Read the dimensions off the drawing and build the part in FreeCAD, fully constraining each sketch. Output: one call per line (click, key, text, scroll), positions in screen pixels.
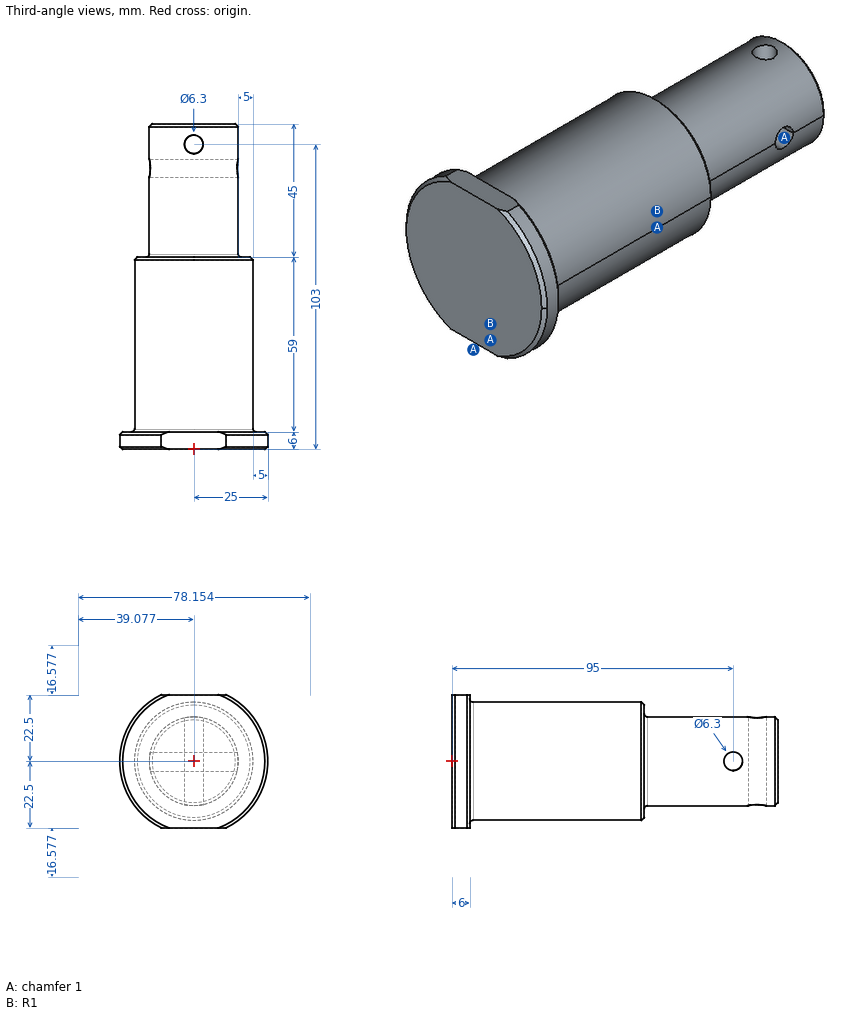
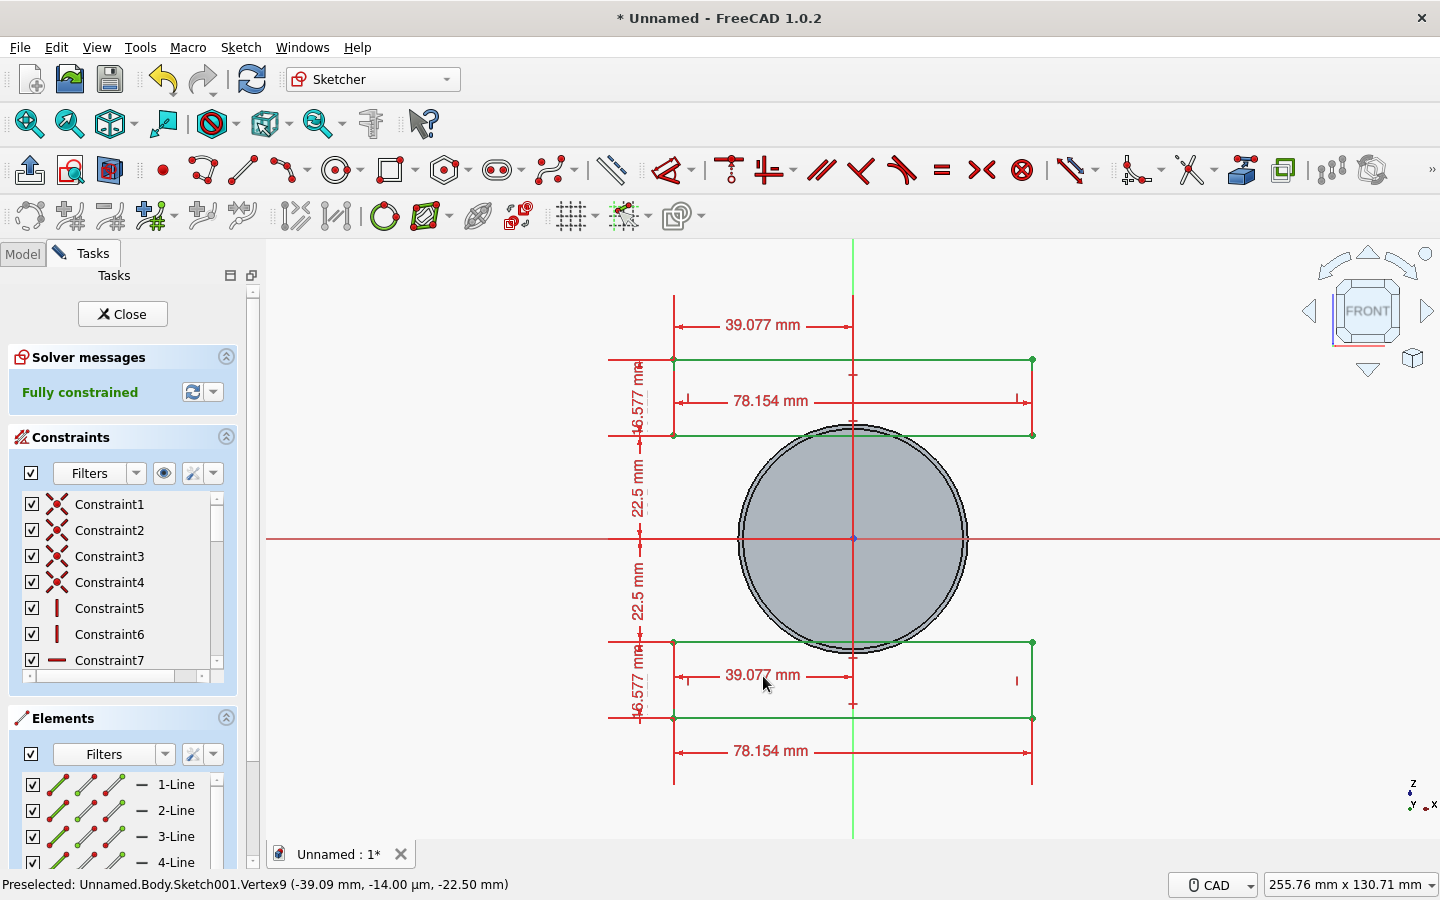
click(123, 314)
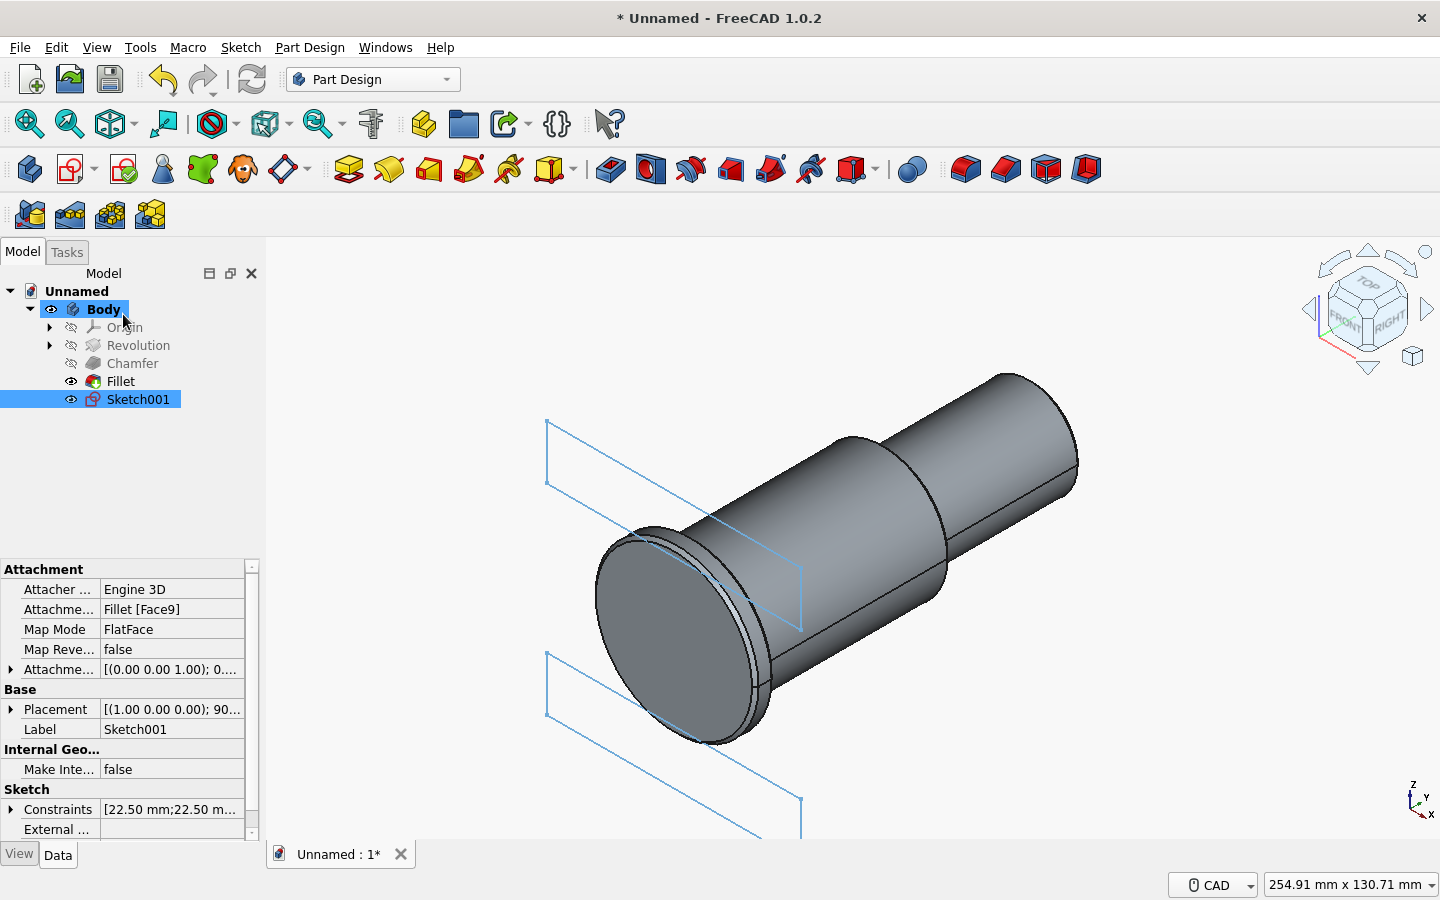
click(612, 170)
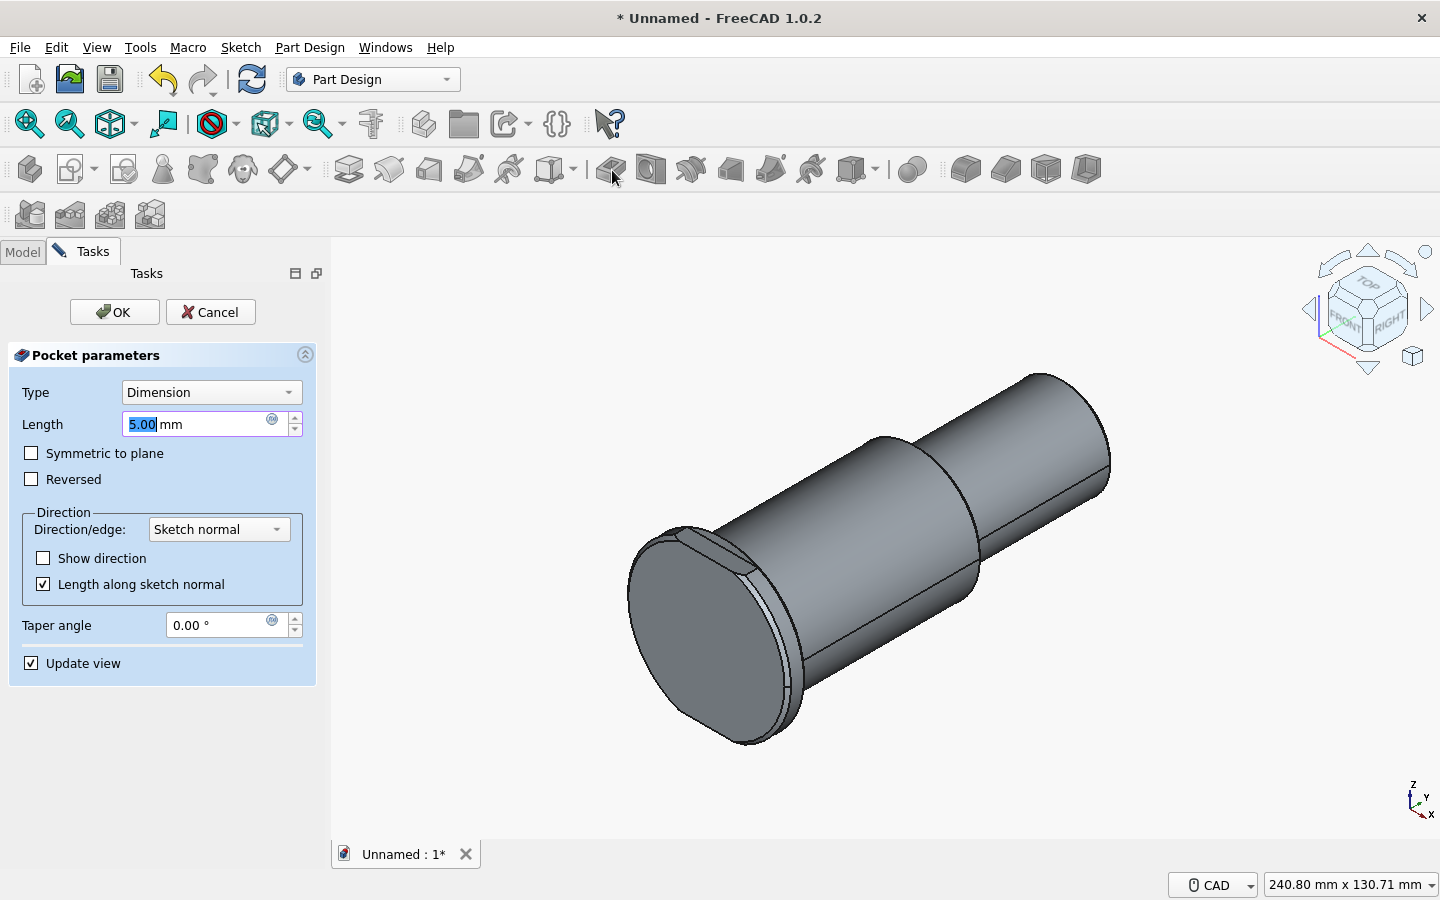
text(6)
key(Tab)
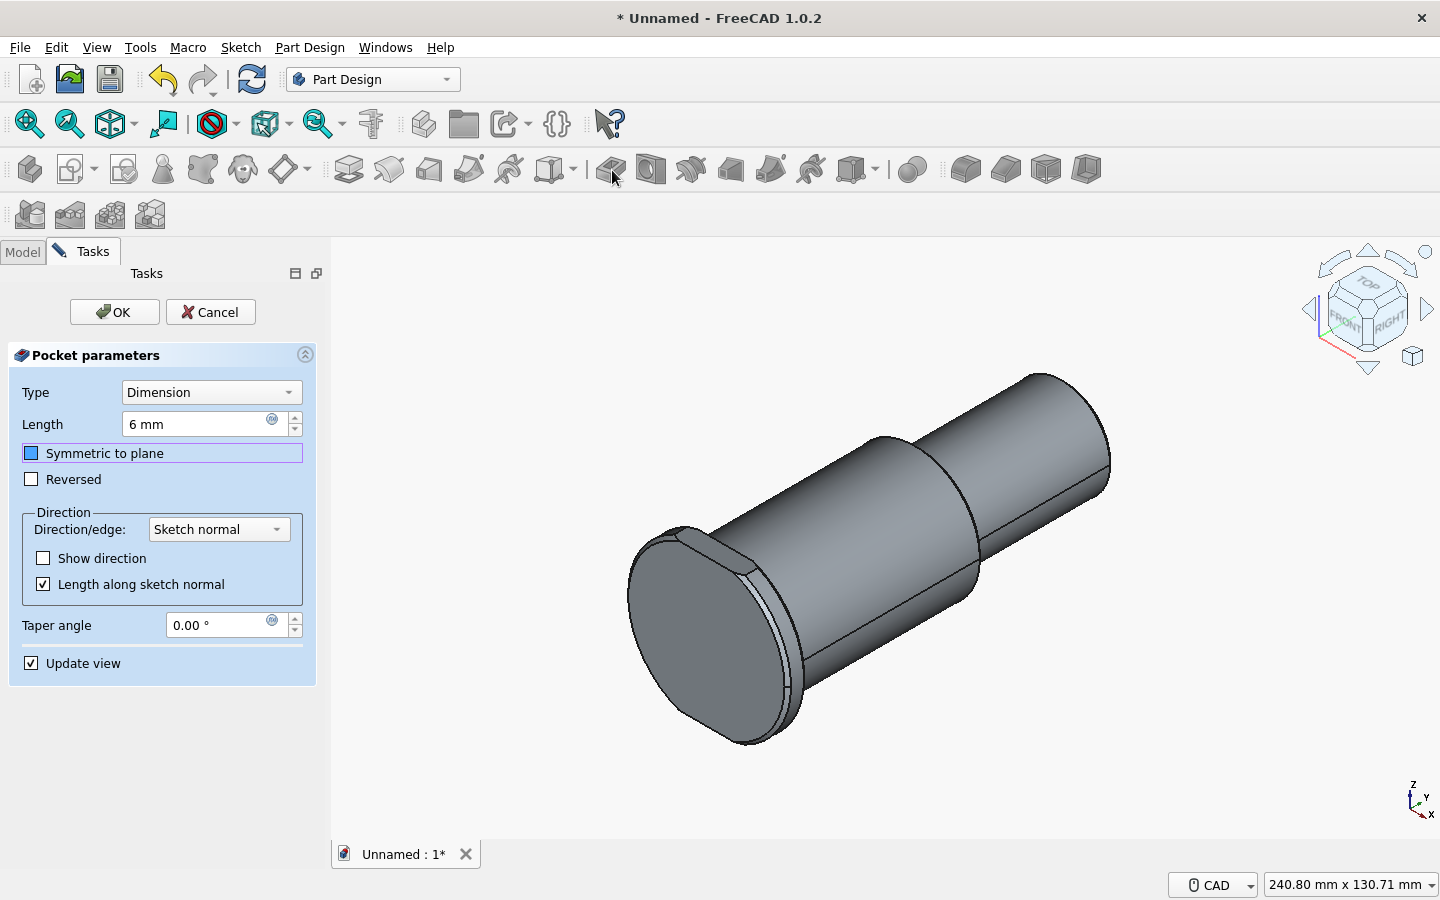
click(115, 312)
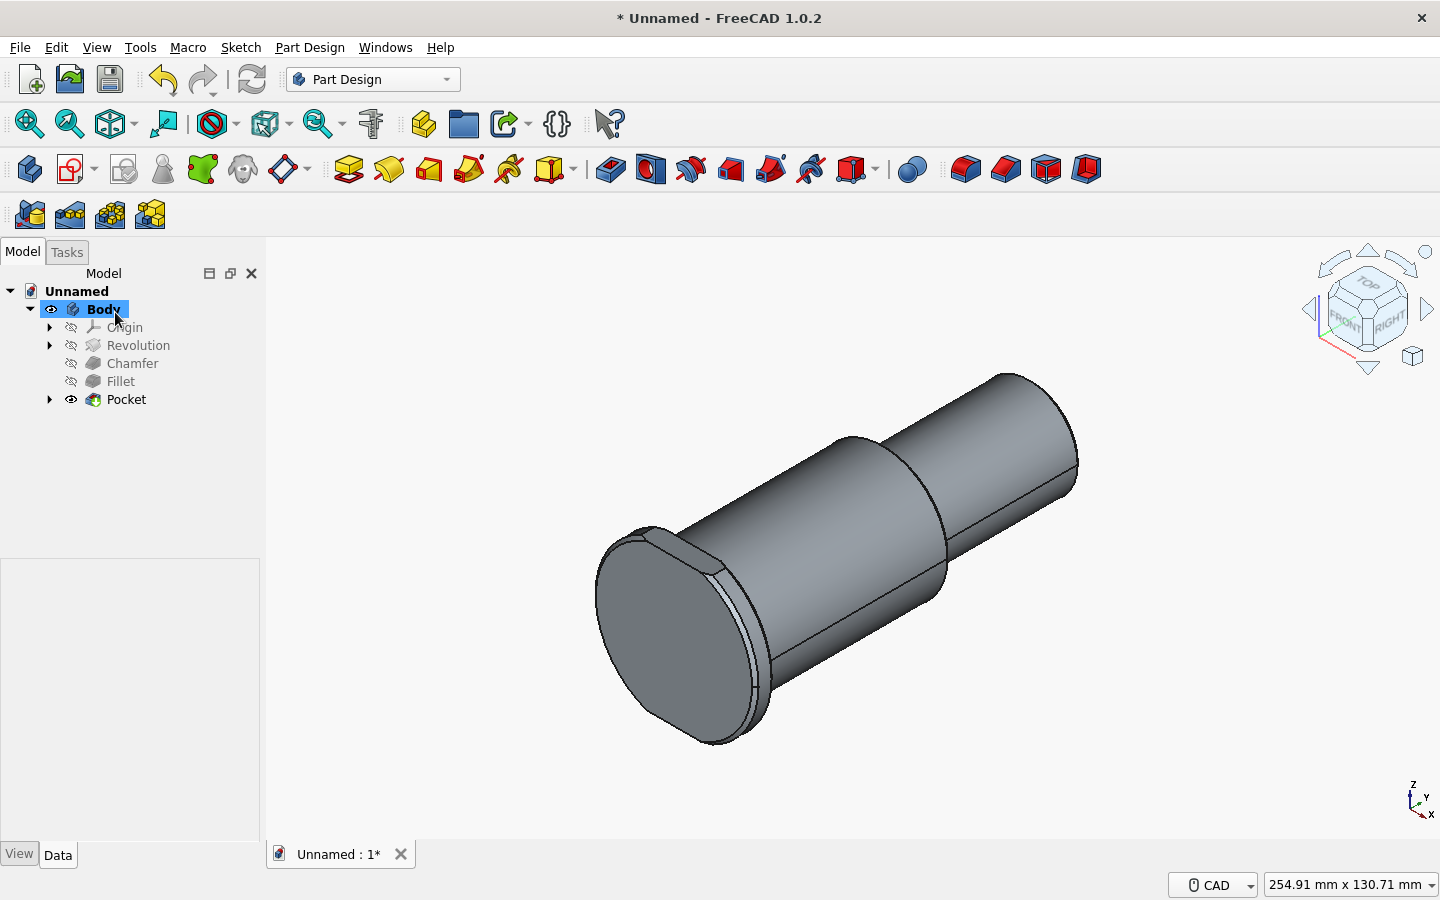
click(70, 170)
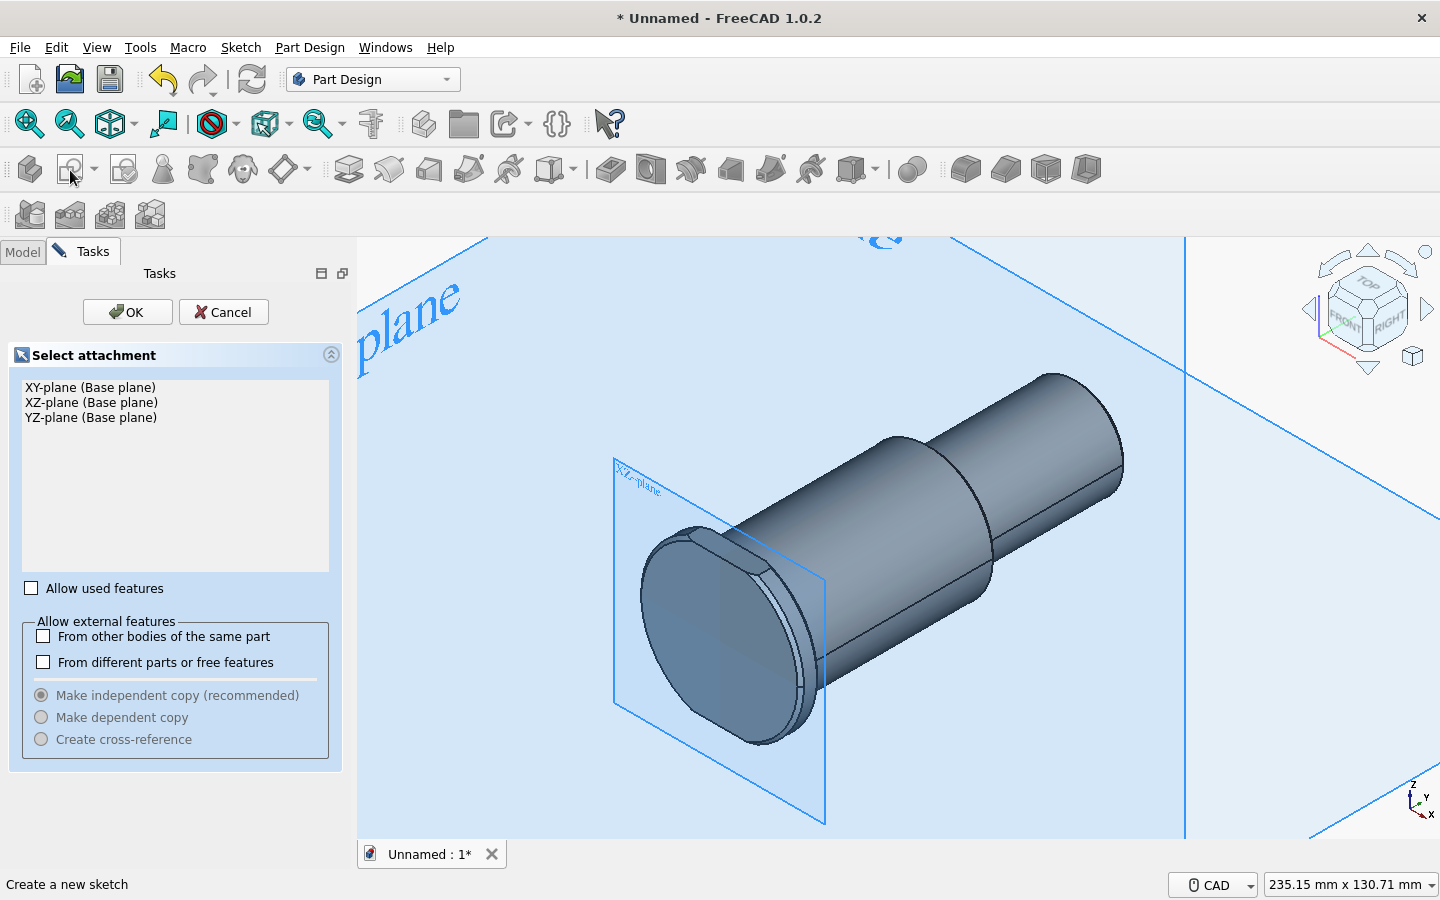
click(82, 388)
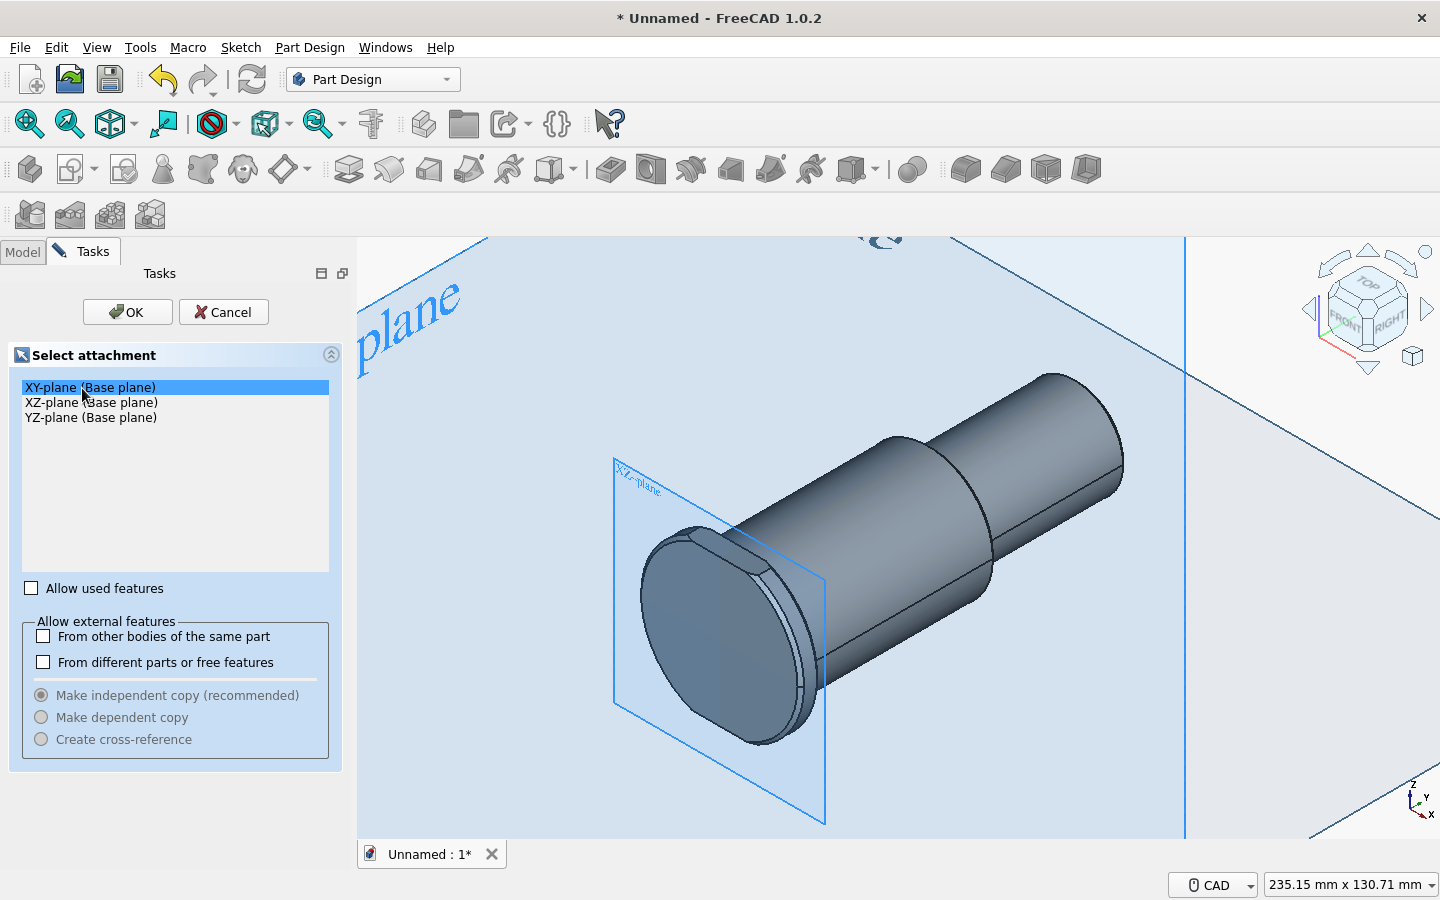
click(128, 312)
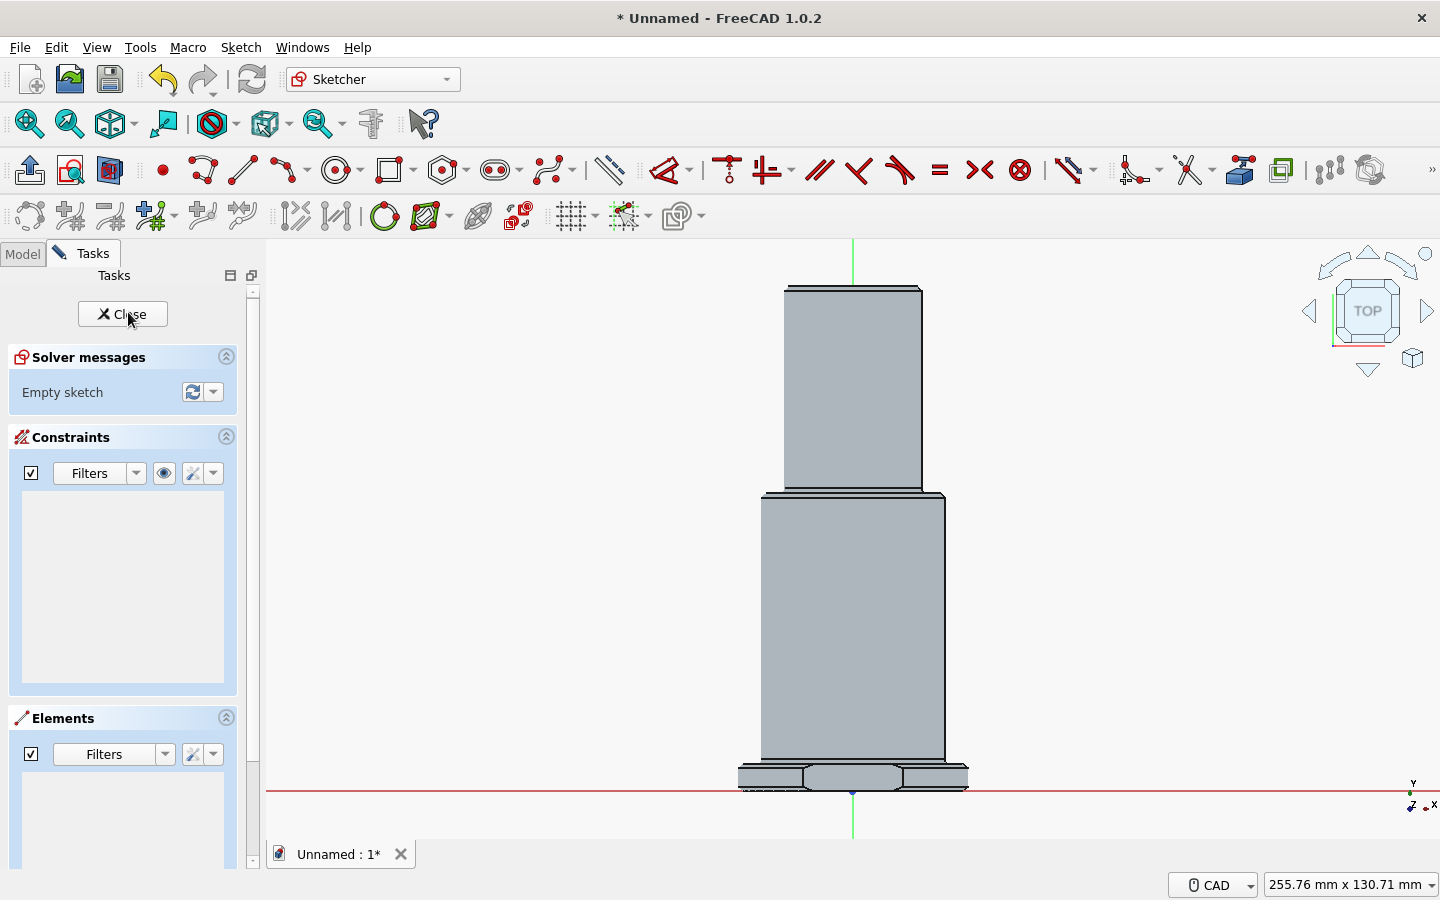
key(q)
key(s)